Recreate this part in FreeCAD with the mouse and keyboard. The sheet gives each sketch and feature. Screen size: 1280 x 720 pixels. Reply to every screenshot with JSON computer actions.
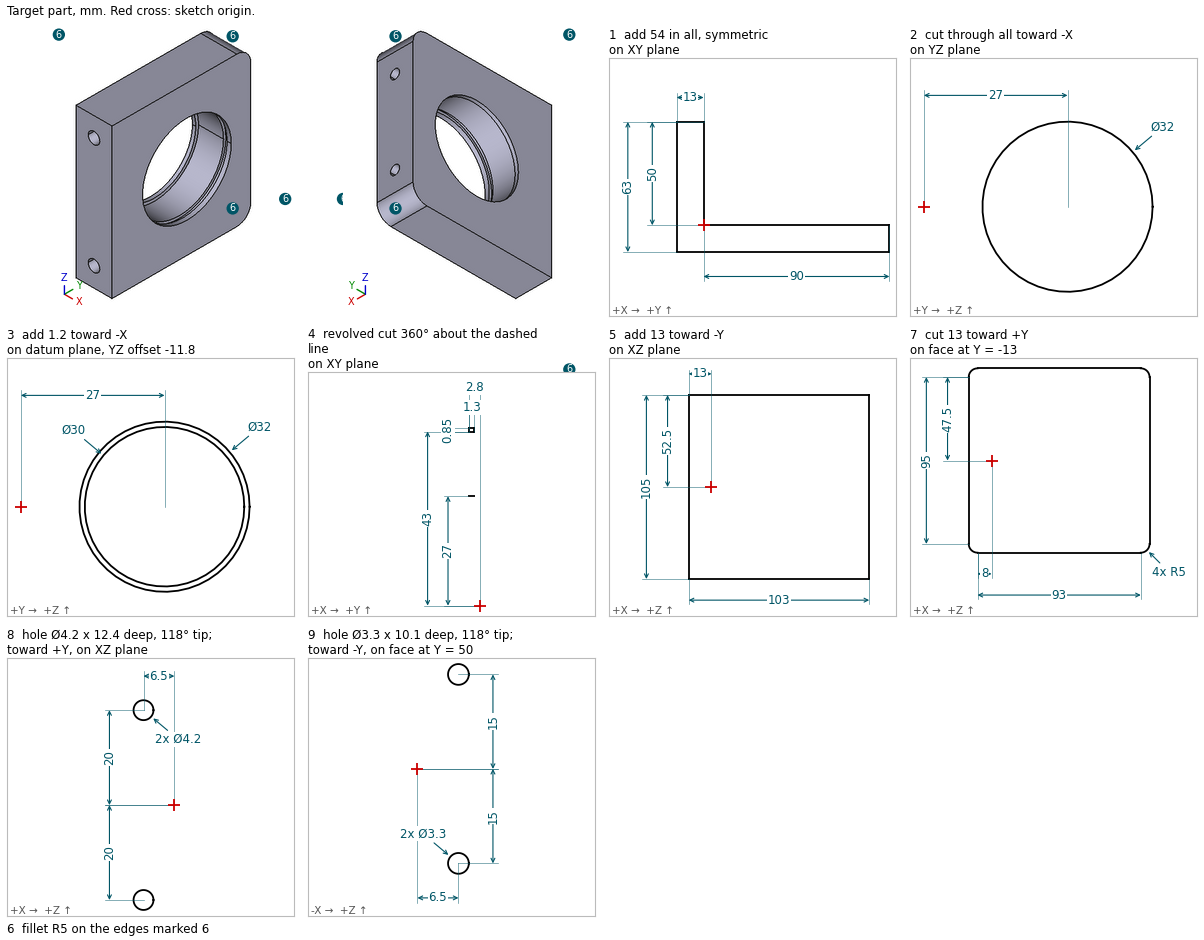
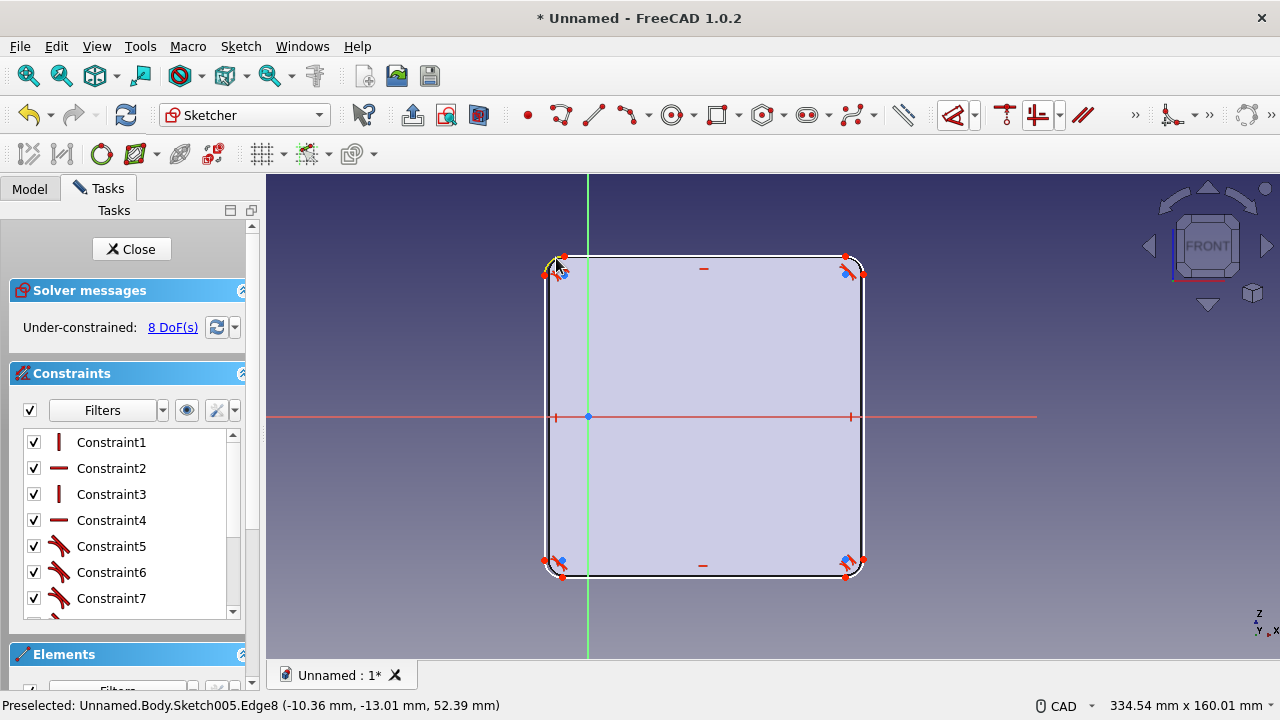
{"action": "scroll", "coordinate": [547, 568], "scroll_direction": "up", "scroll_amount": 3}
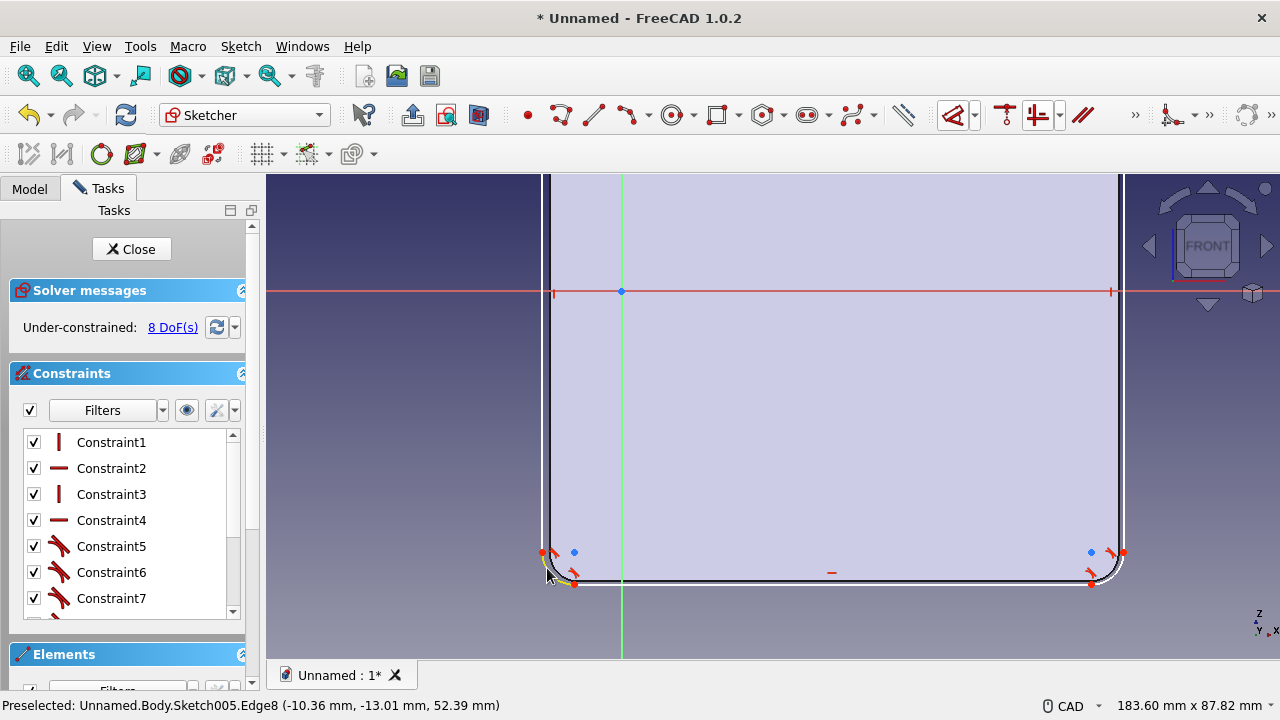
{"action": "left_click", "coordinate": [546, 567]}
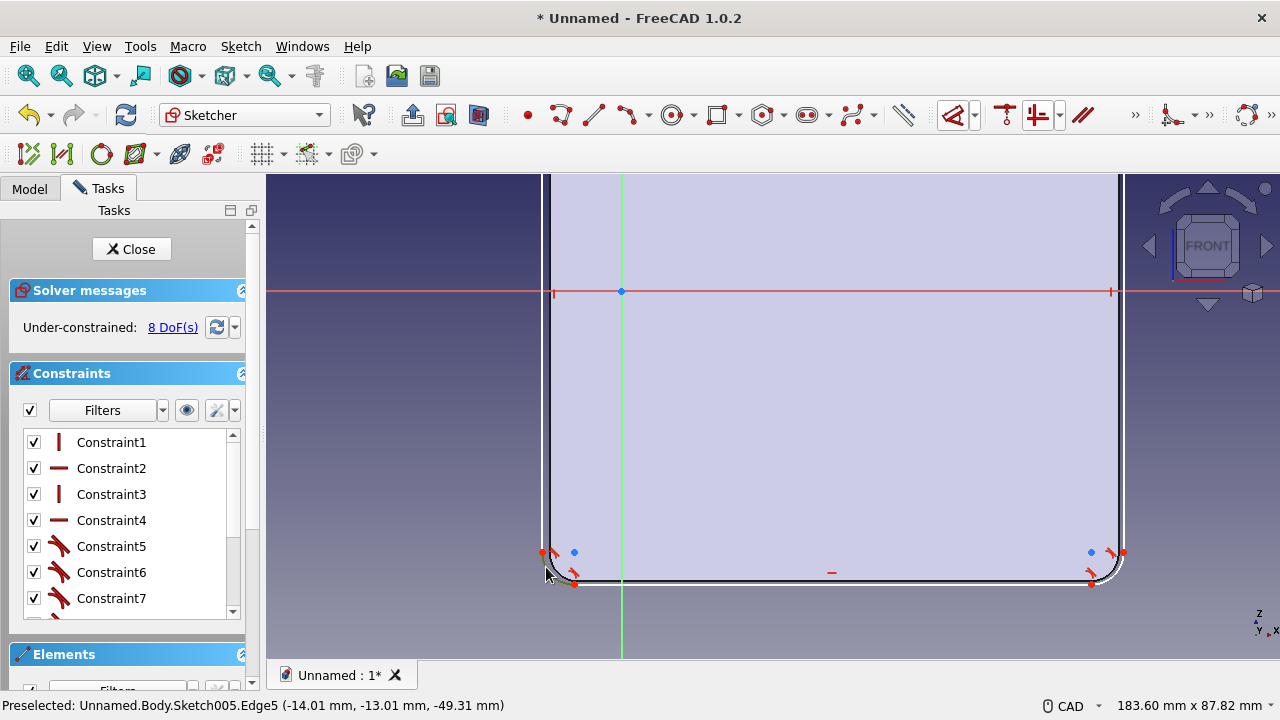
{"action": "left_click", "coordinate": [1106, 581]}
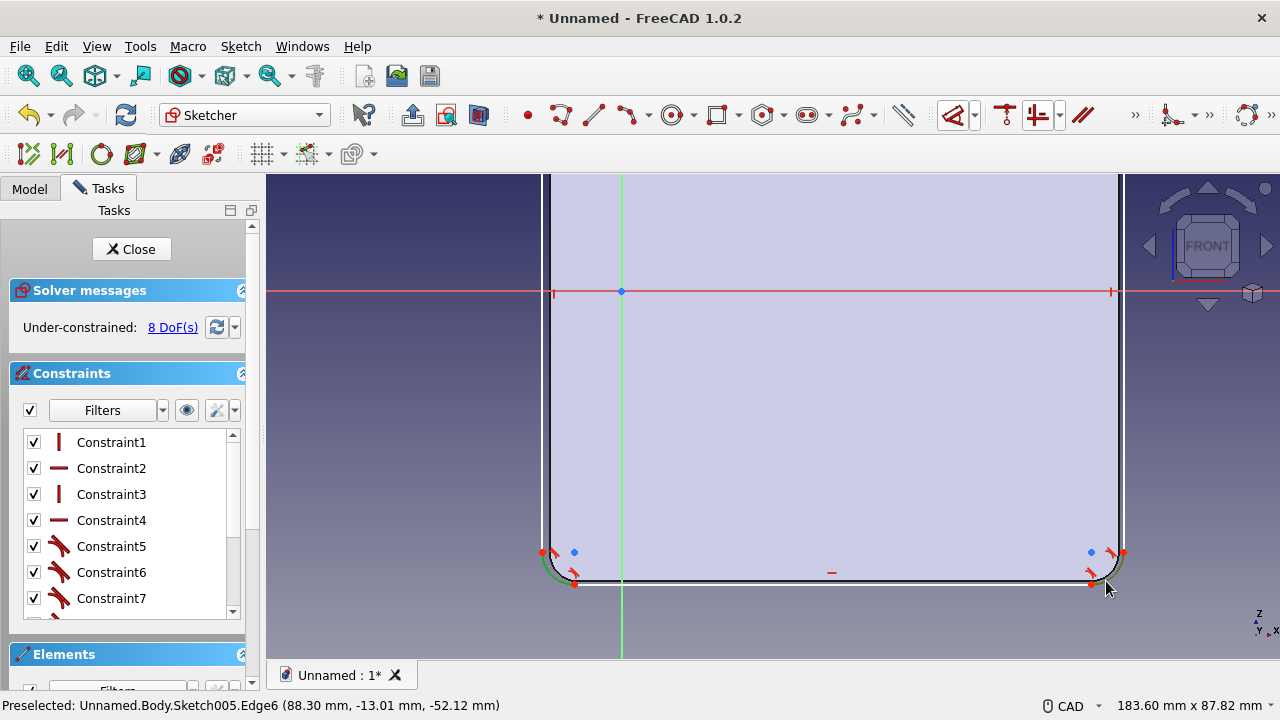
{"action": "scroll", "coordinate": [547, 569], "scroll_direction": "down", "scroll_amount": 3}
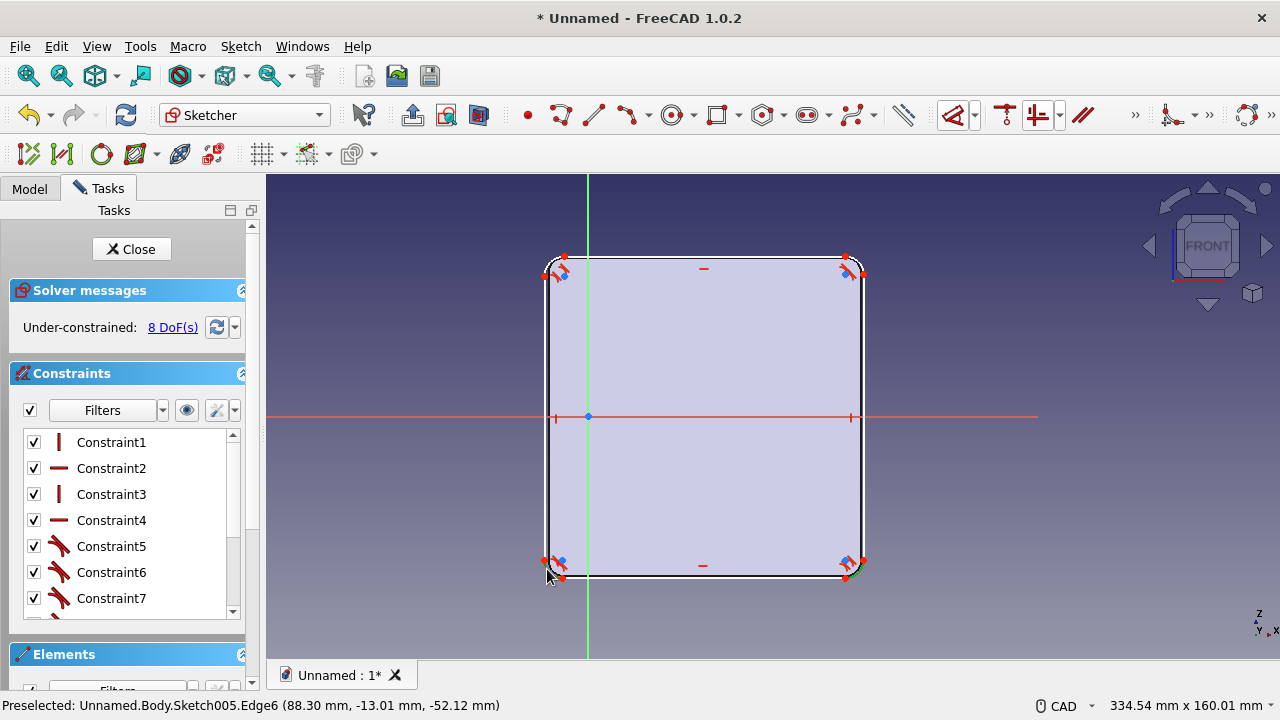
{"action": "scroll", "coordinate": [862, 266], "scroll_direction": "up", "scroll_amount": 3}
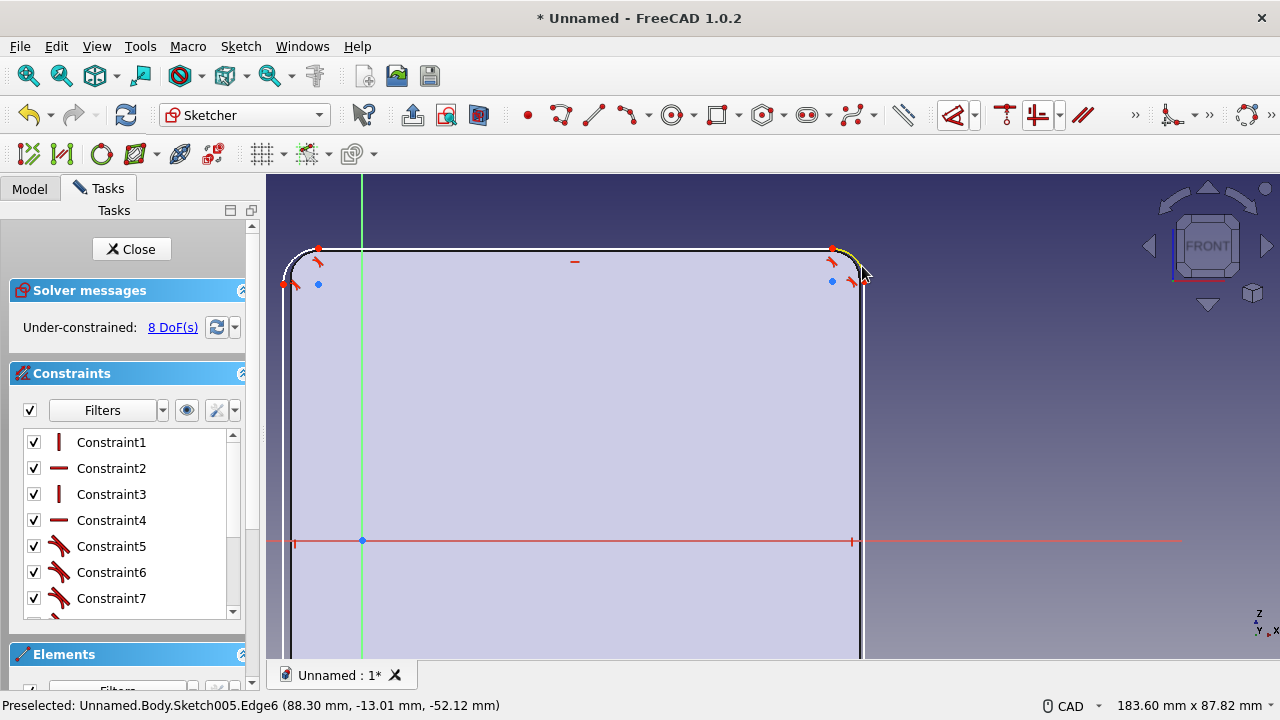
{"action": "left_click", "coordinate": [861, 267]}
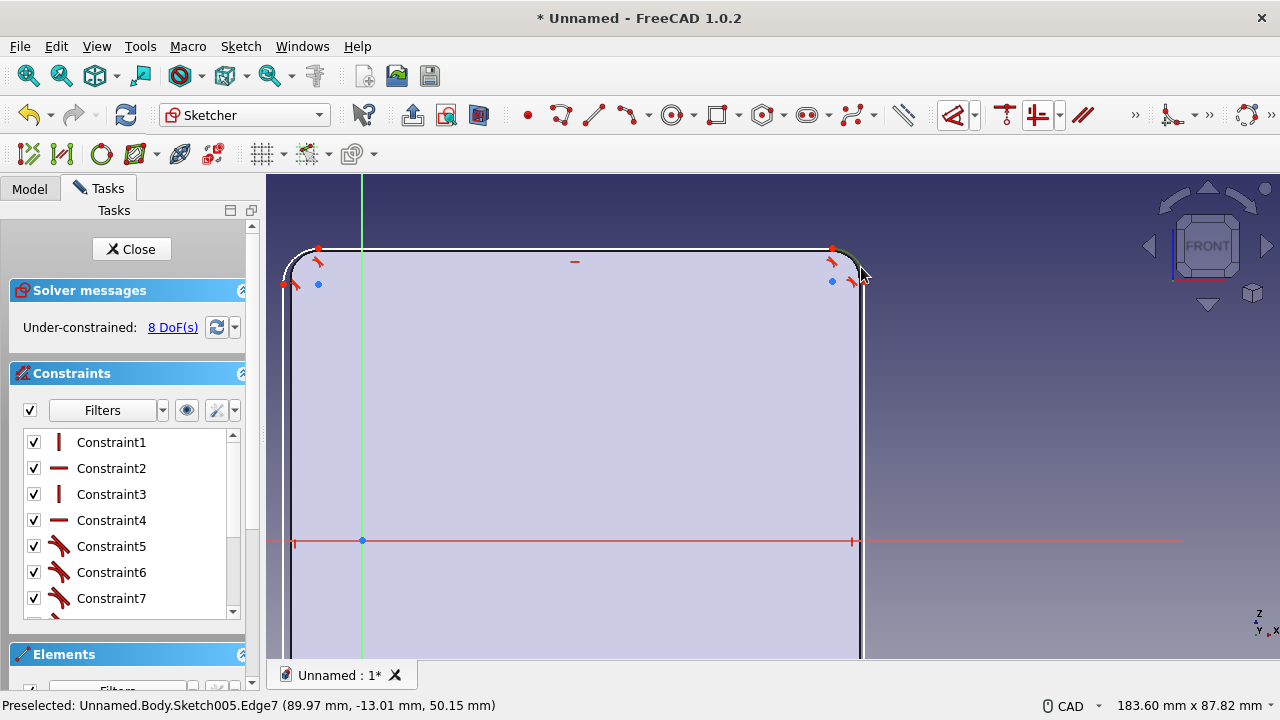
{"action": "left_click", "coordinate": [303, 253]}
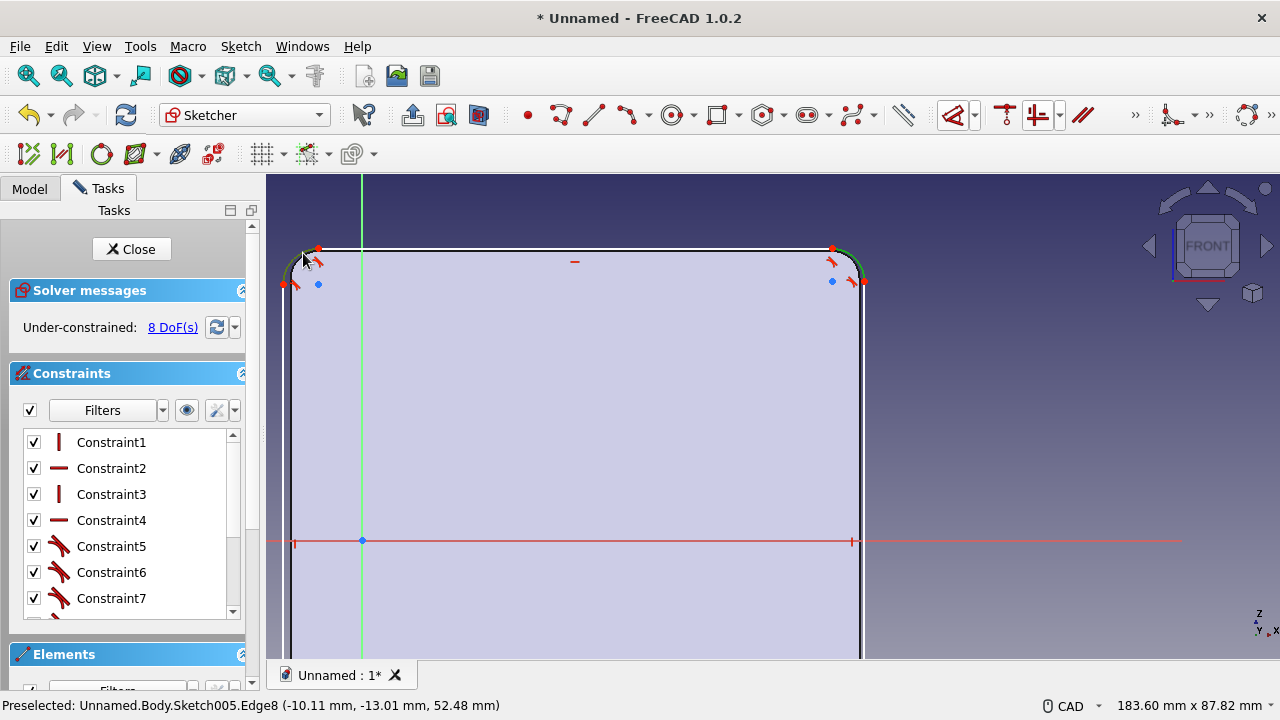
{"action": "key", "text": "e"}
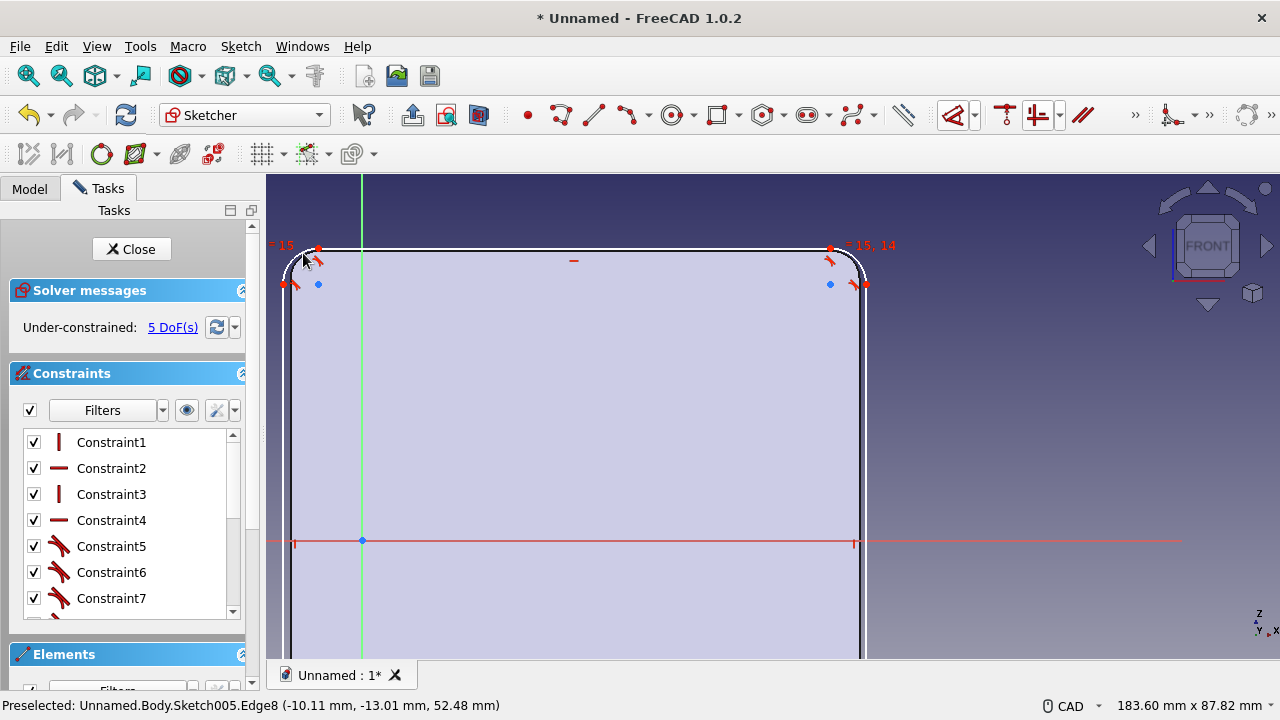
{"action": "scroll", "coordinate": [862, 265], "scroll_direction": "down", "scroll_amount": 3}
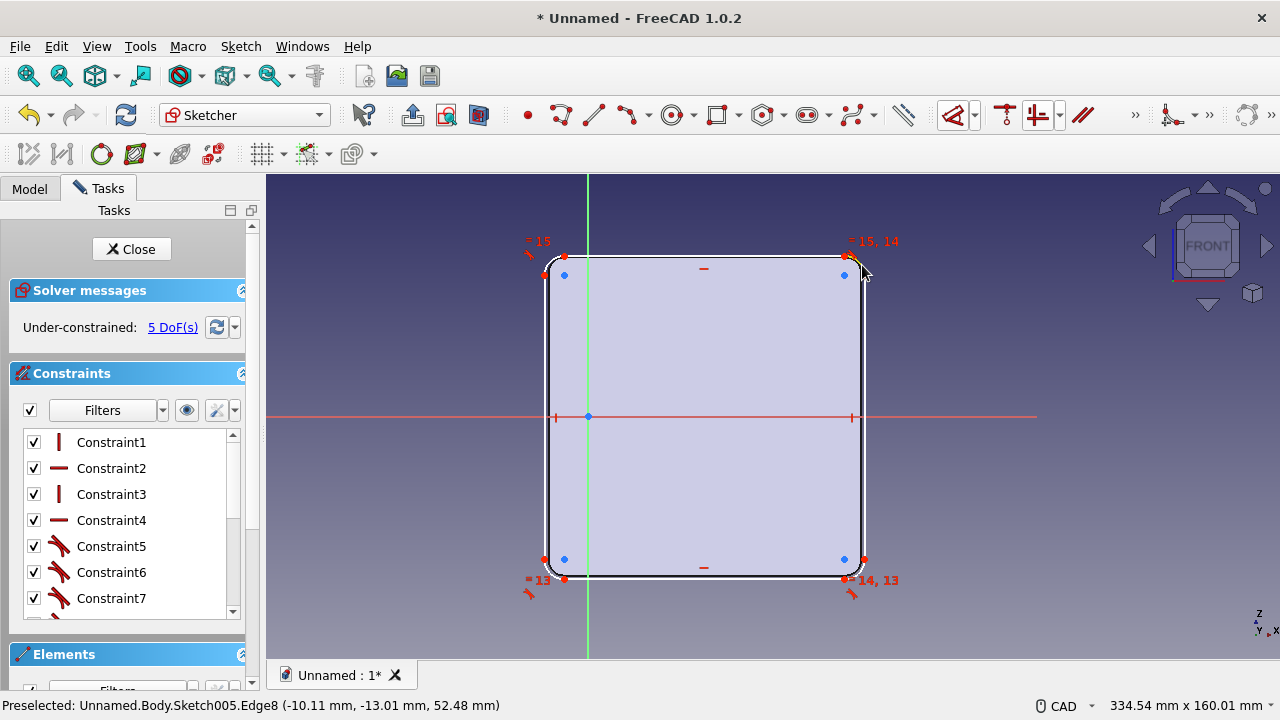
{"action": "scroll", "coordinate": [547, 569], "scroll_direction": "up", "scroll_amount": 5}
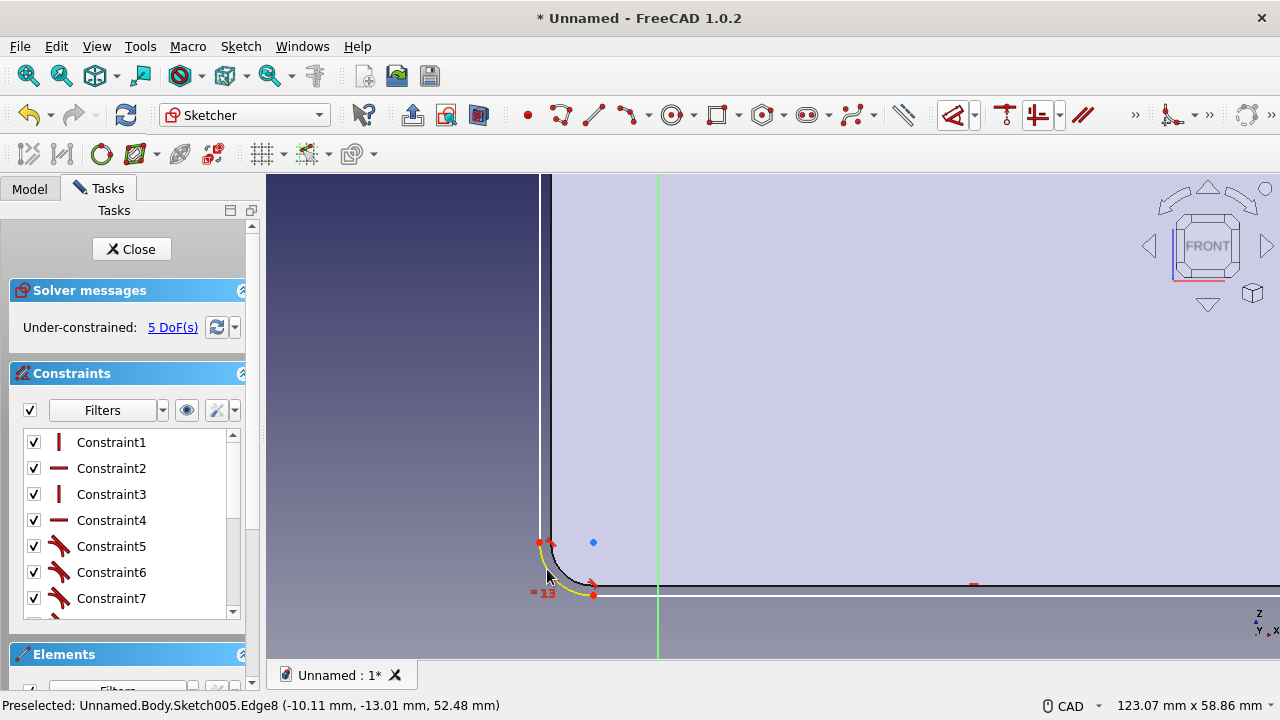
{"action": "left_click", "coordinate": [546, 566]}